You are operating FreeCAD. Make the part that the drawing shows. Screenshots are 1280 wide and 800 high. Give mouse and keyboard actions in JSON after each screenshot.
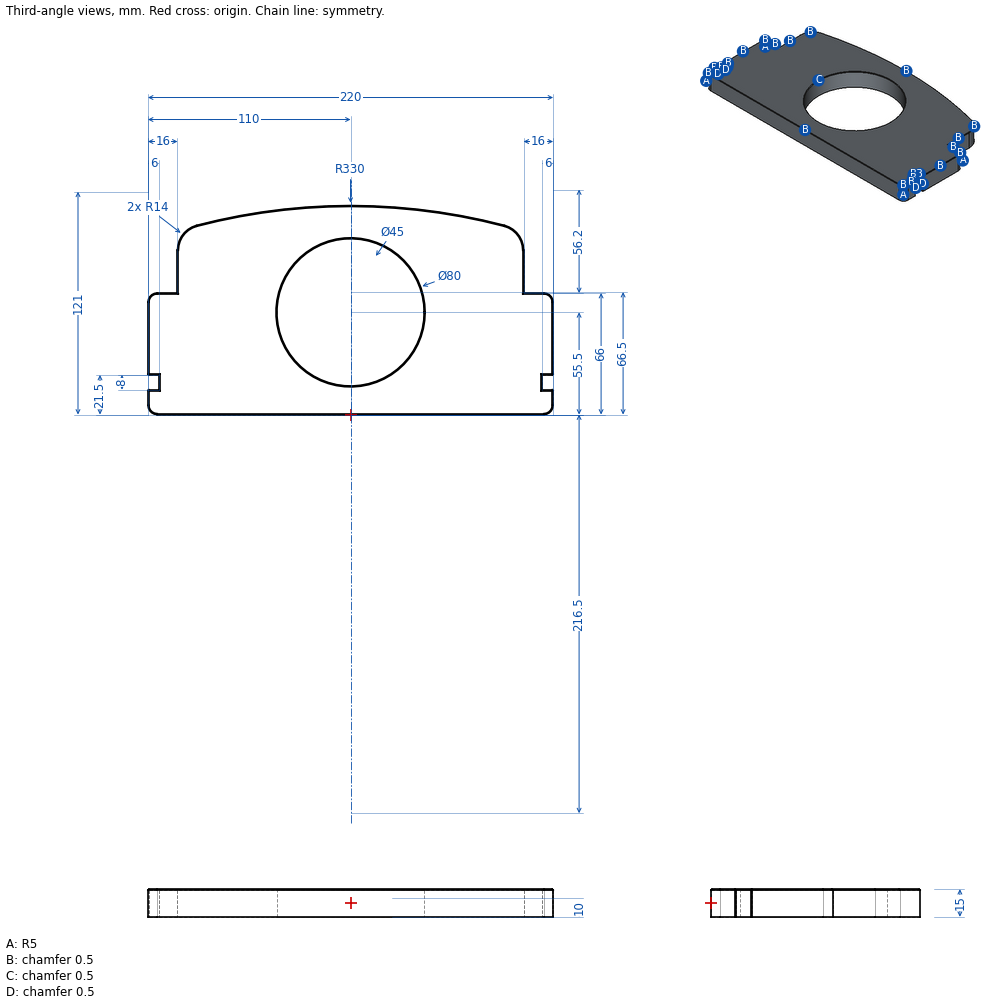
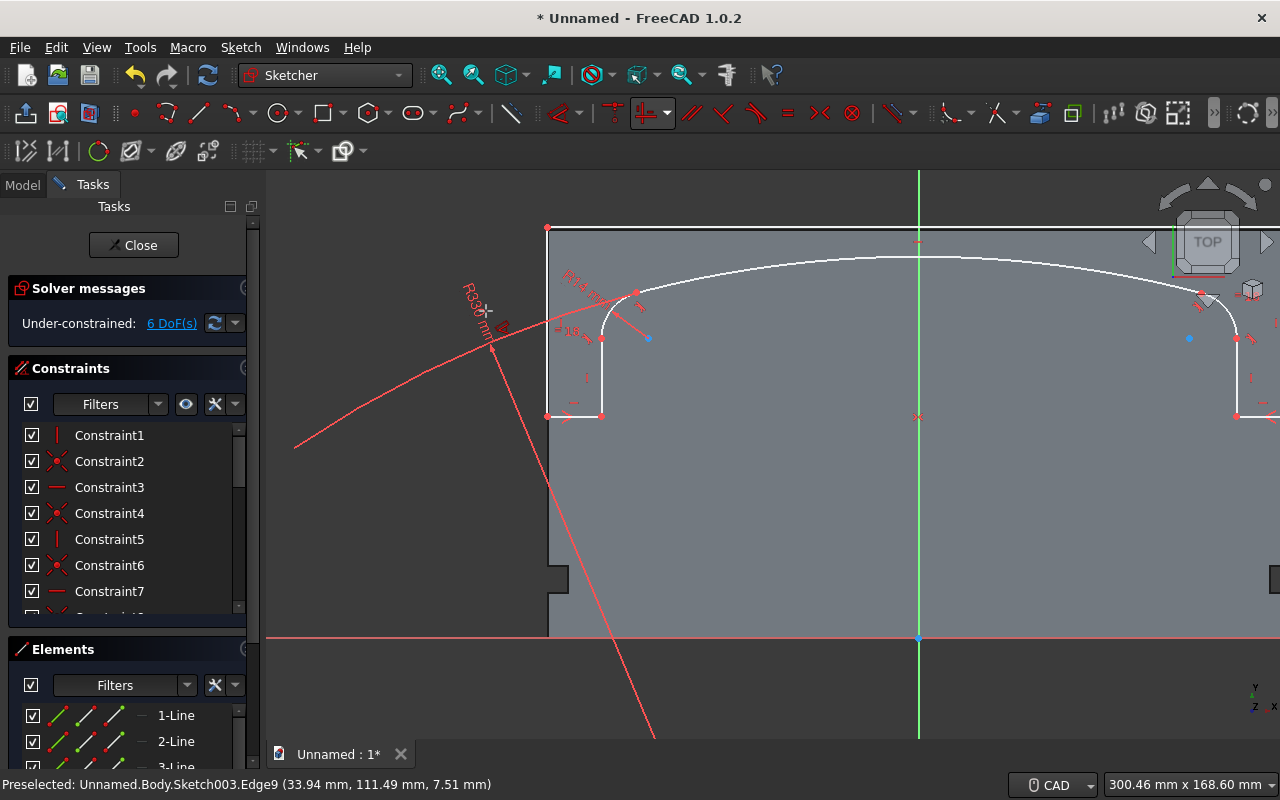
{"action": "scroll", "coordinate": [294, 500], "scroll_direction": "down", "scroll_amount": 2}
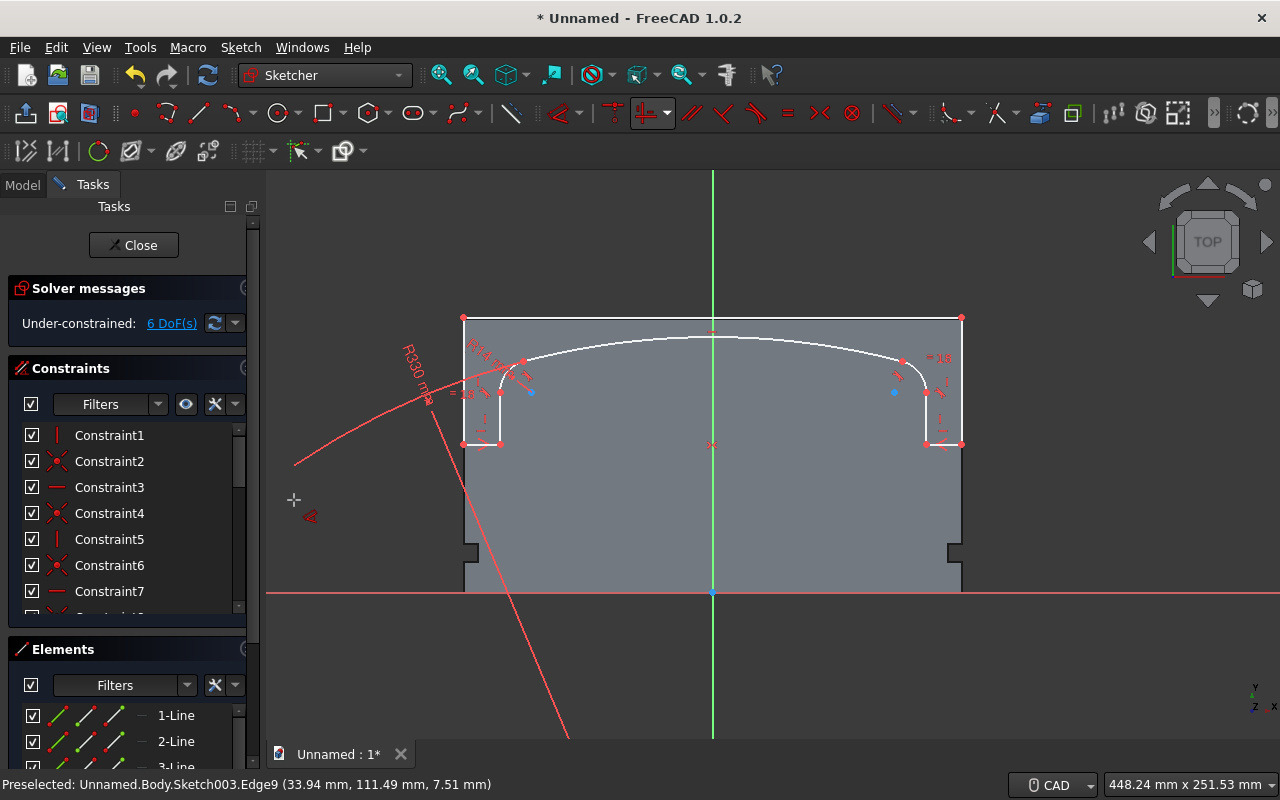
{"action": "scroll", "coordinate": [937, 445], "scroll_direction": "up", "scroll_amount": 2}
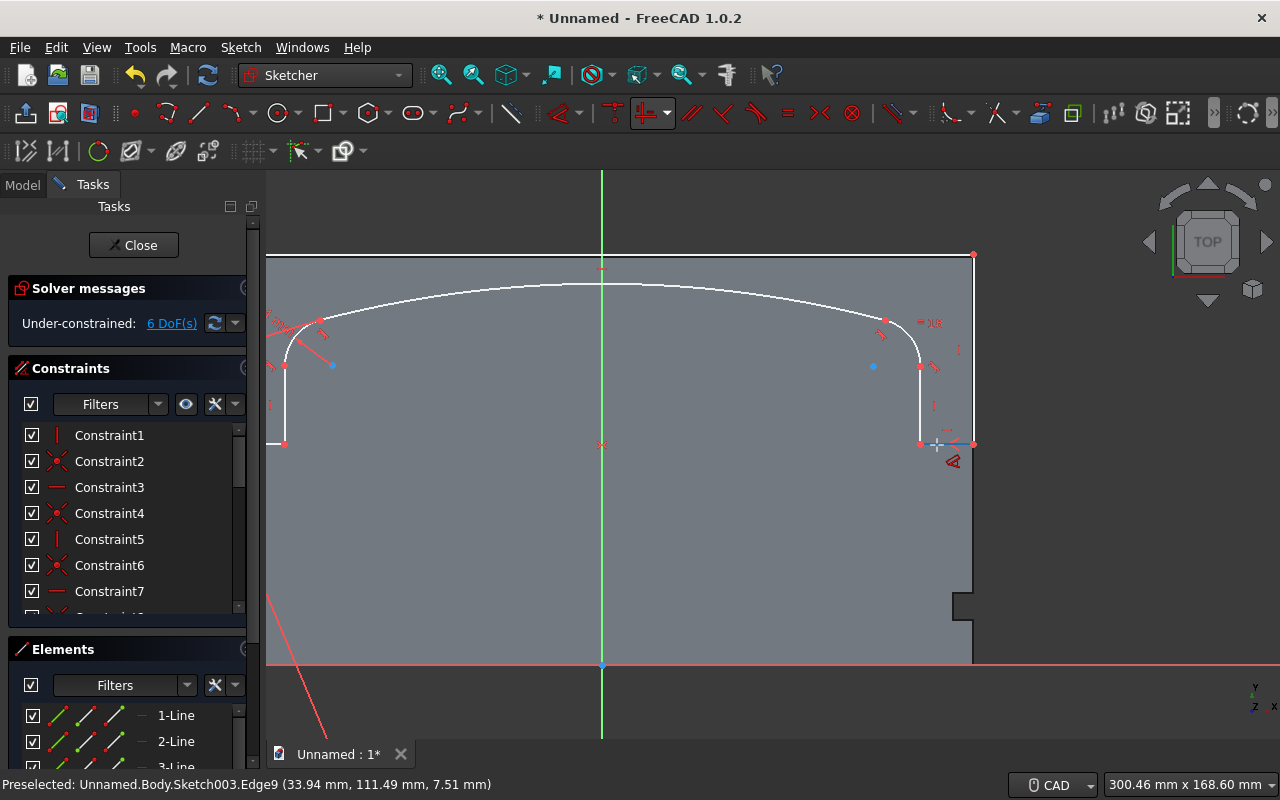
{"action": "left_click", "coordinate": [936, 444]}
{"action": "left_click", "coordinate": [947, 410]}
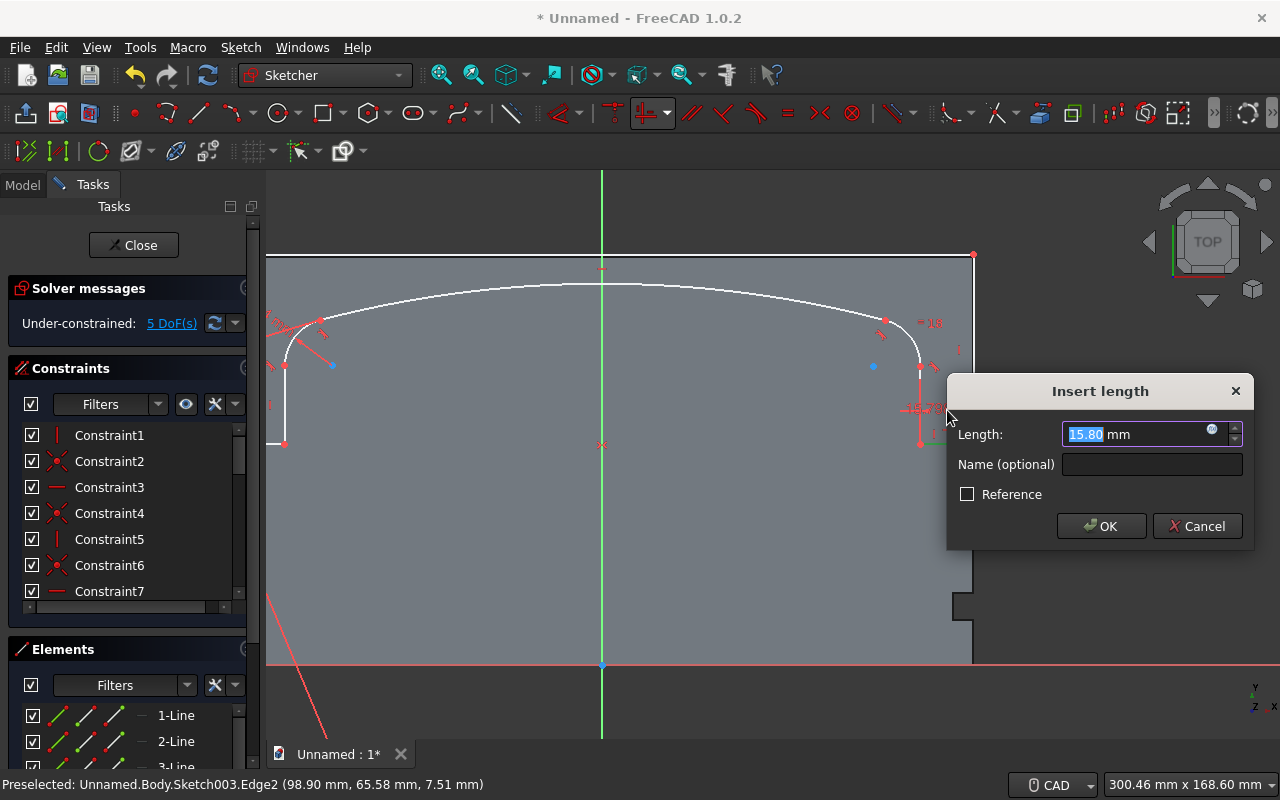
{"action": "type", "text": "16"}
{"action": "key", "text": "Return"}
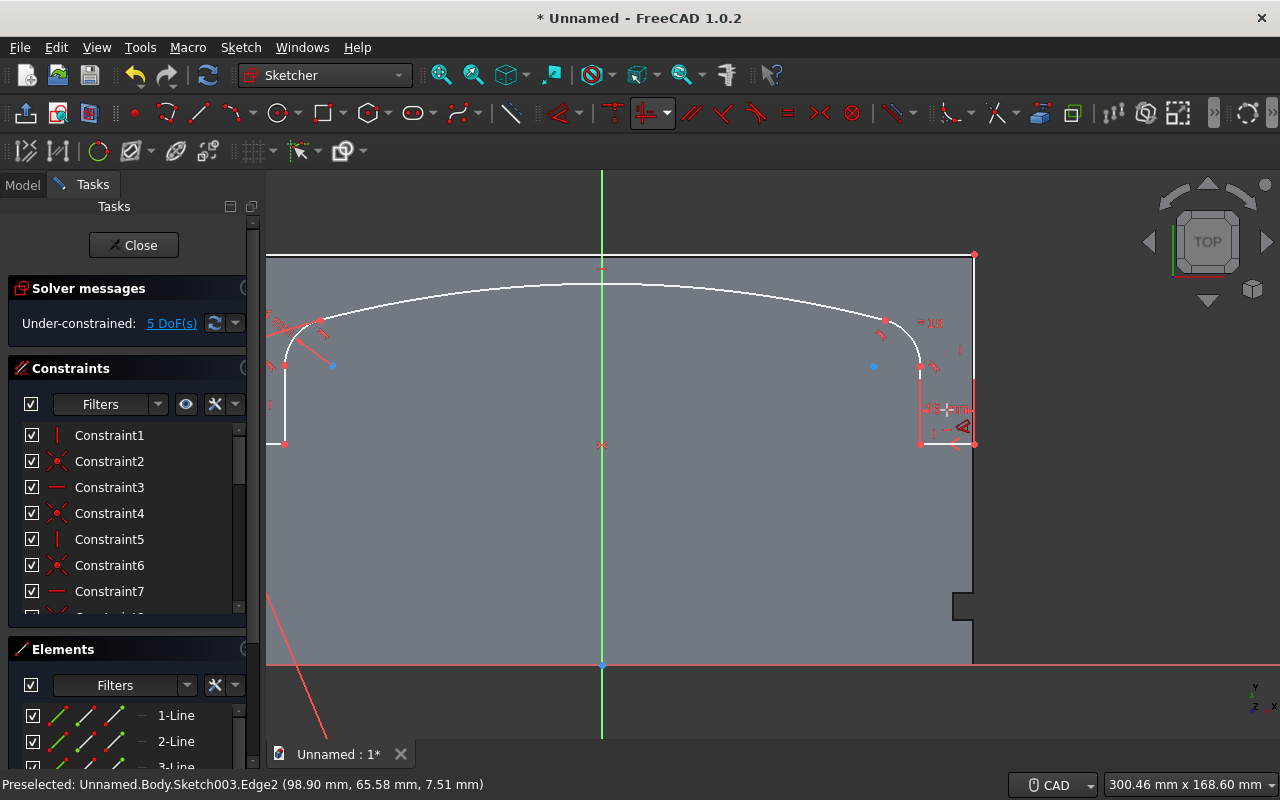
{"action": "scroll", "coordinate": [1115, 433], "scroll_direction": "down", "scroll_amount": 1}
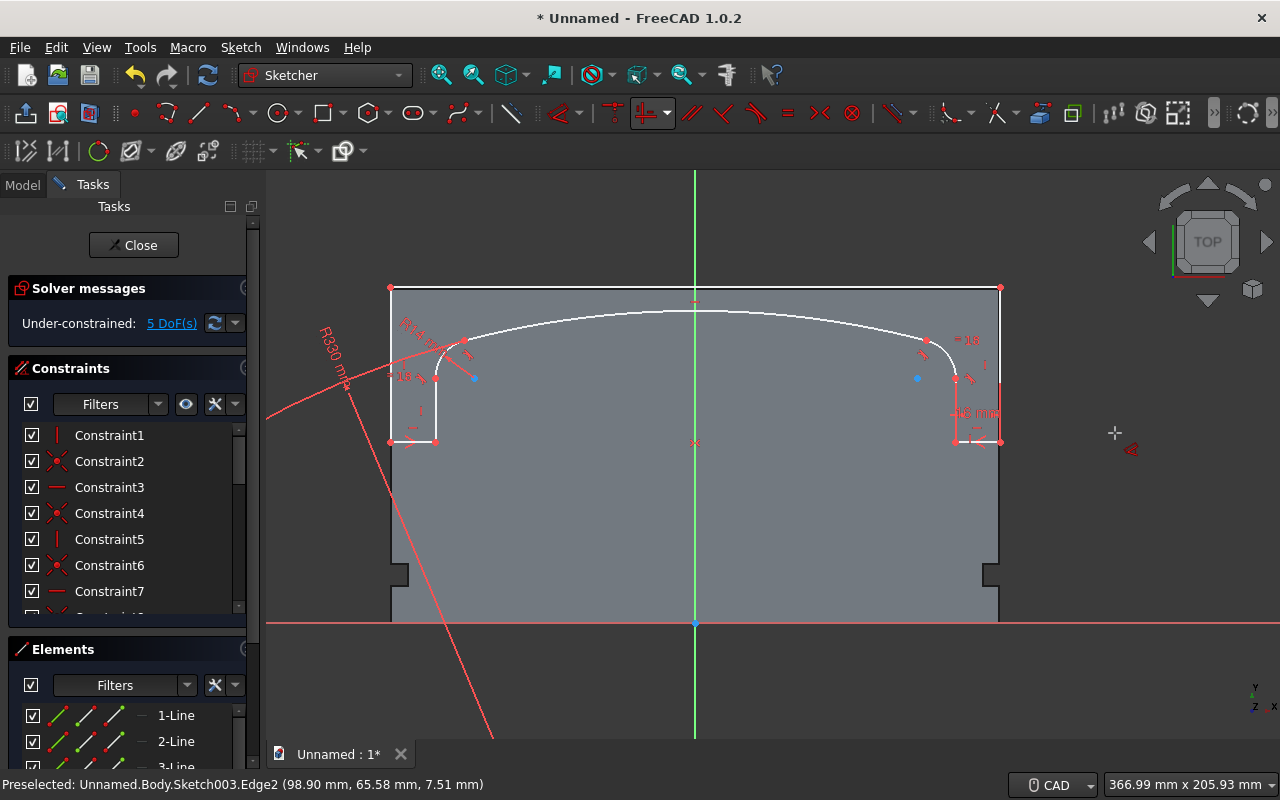
{"action": "left_click", "coordinate": [404, 442]}
{"action": "left_click", "coordinate": [413, 408]}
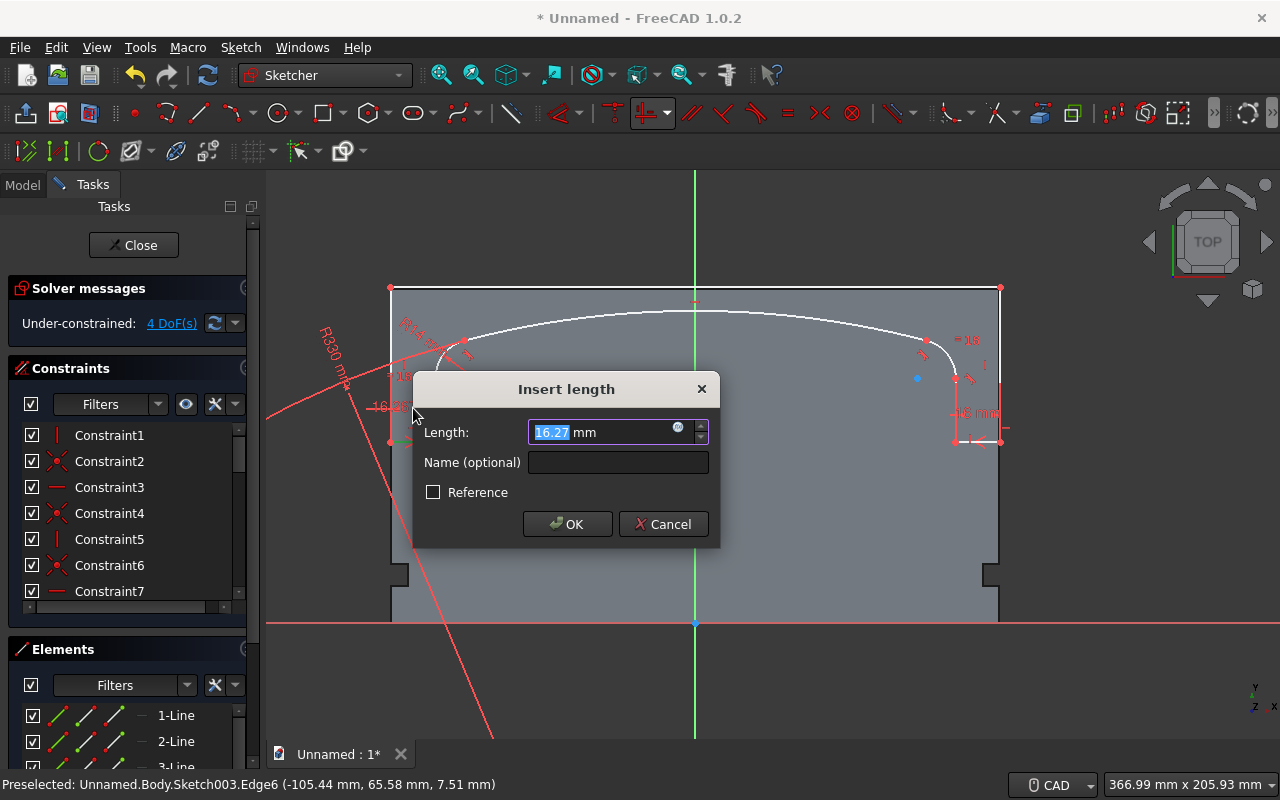
{"action": "type", "text": "16"}
{"action": "key", "text": "Return"}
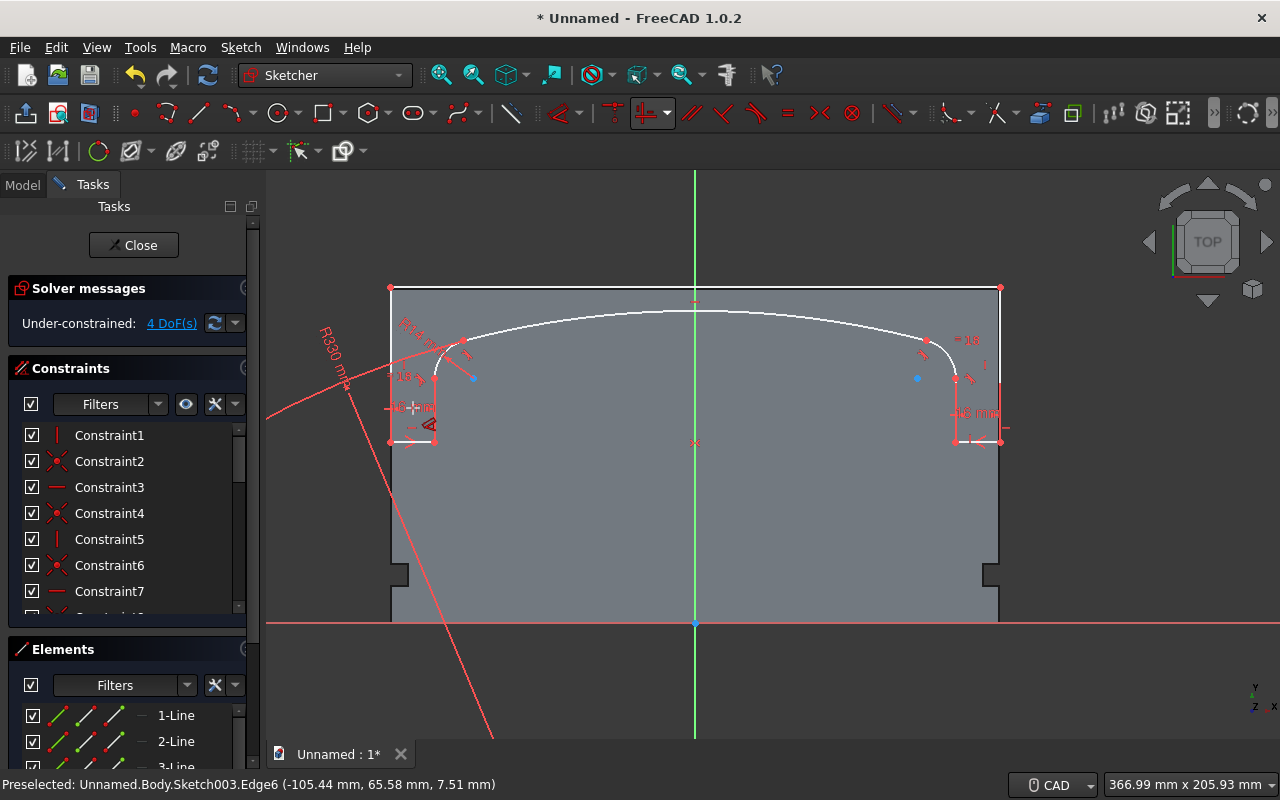
{"action": "left_click", "coordinate": [817, 287]}
{"action": "left_click", "coordinate": [555, 253]}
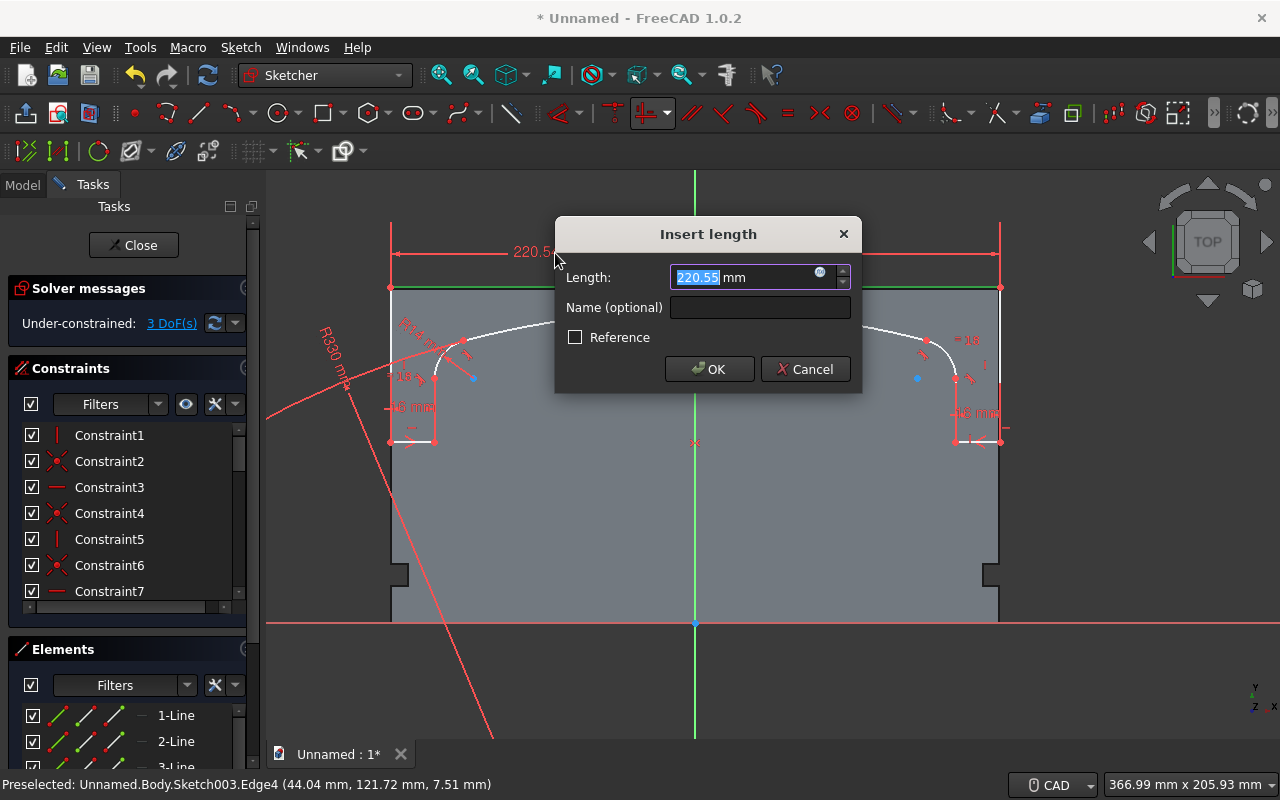
{"action": "type", "text": "220"}
{"action": "key", "text": "Return"}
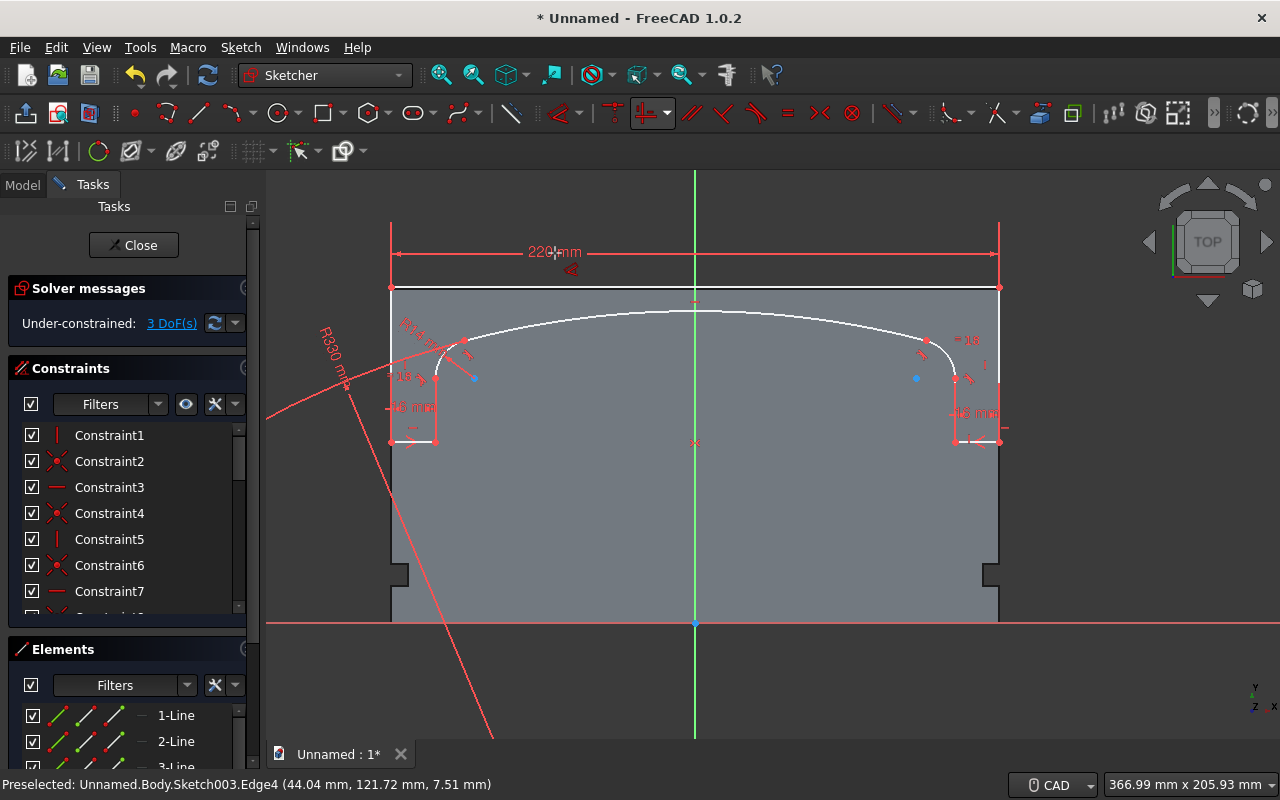
{"action": "left_click", "coordinate": [955, 442]}
{"action": "left_click", "coordinate": [989, 533]}